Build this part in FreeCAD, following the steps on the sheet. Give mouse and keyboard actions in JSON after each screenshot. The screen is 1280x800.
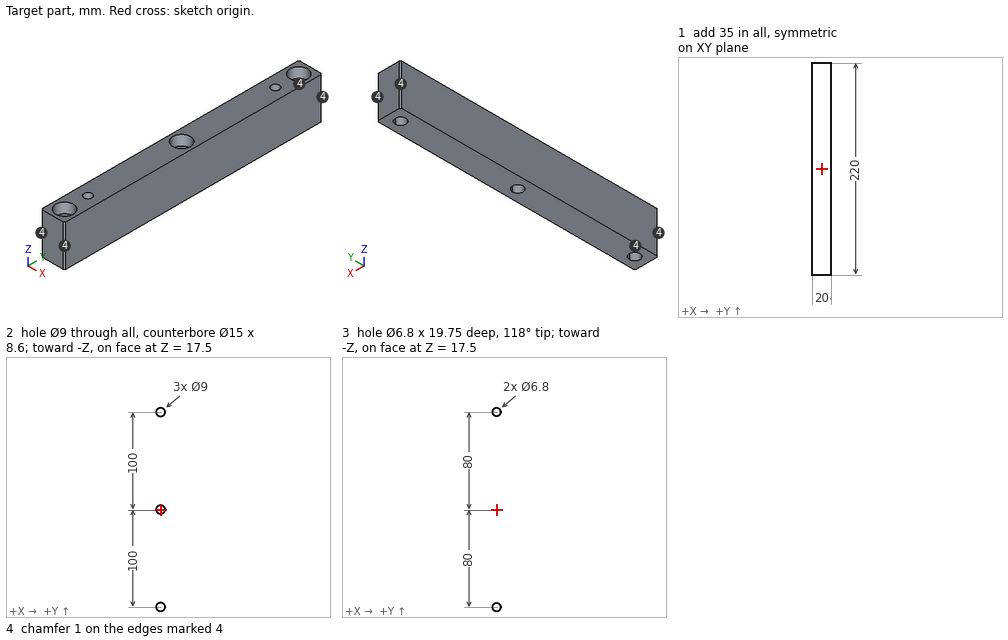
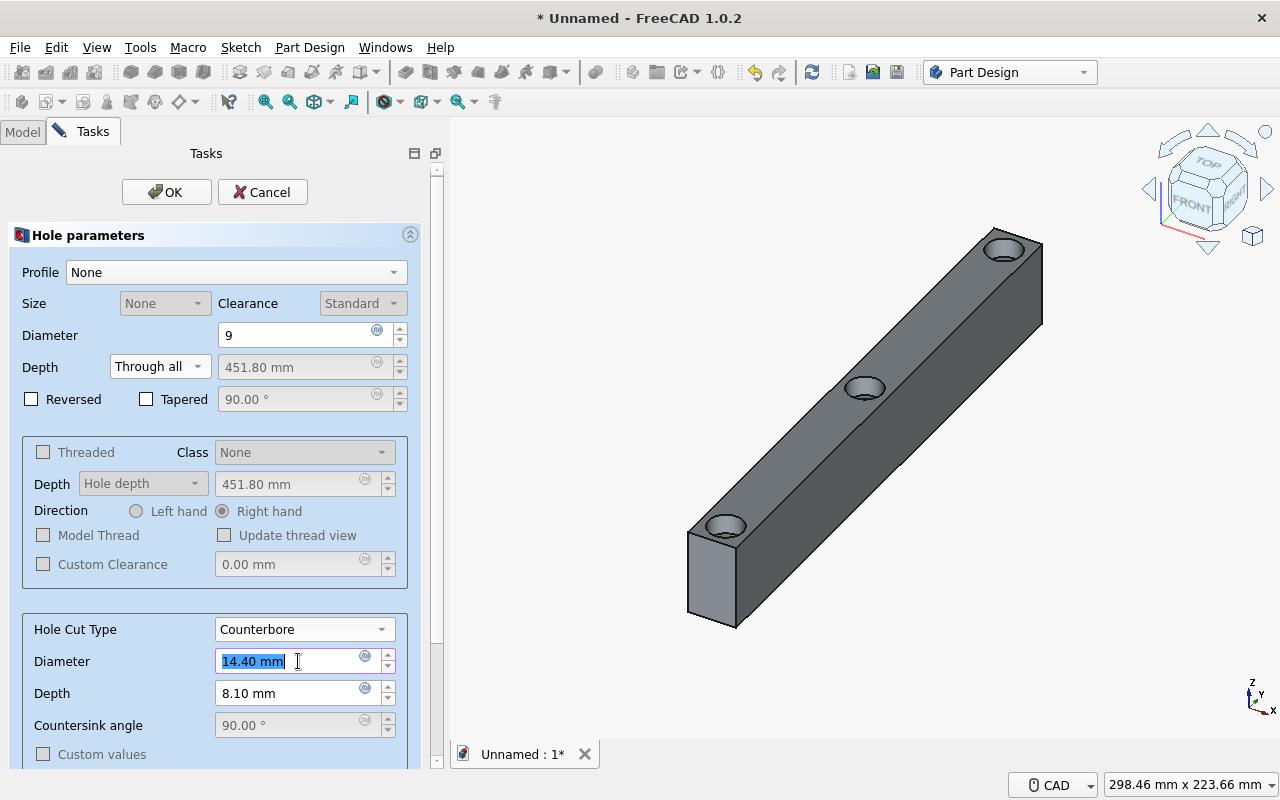
{"action": "type", "text": "15"}
{"action": "key", "text": "Tab"}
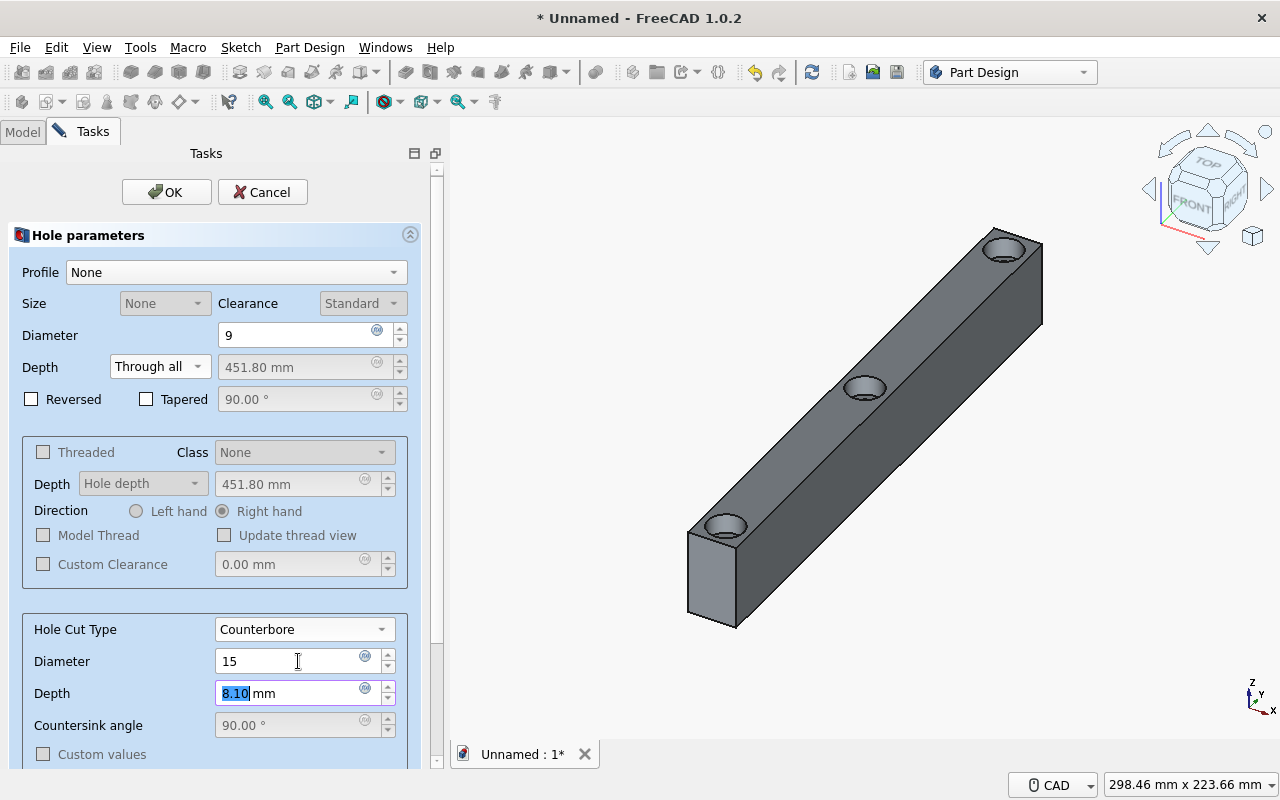
{"action": "type", "text": "8.6"}
{"action": "key", "text": "Tab"}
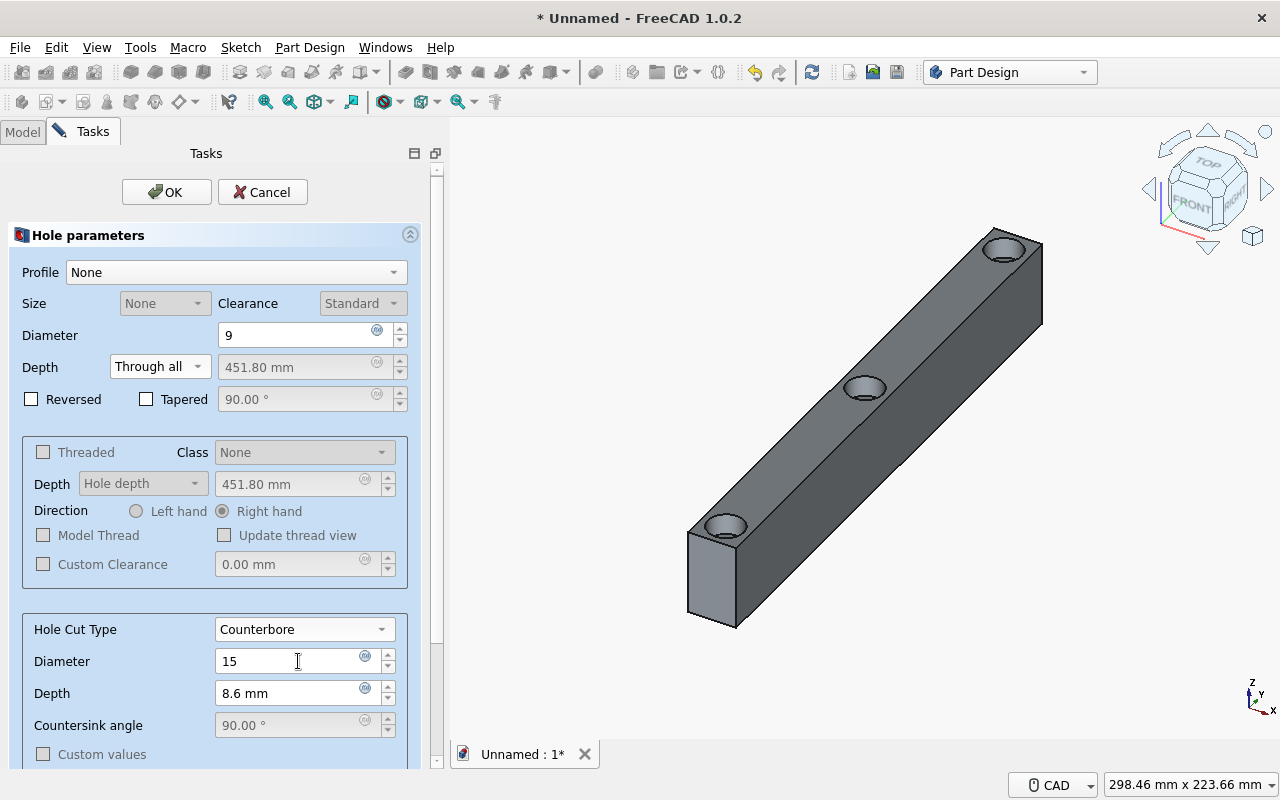
{"action": "left_click", "coordinate": [167, 192]}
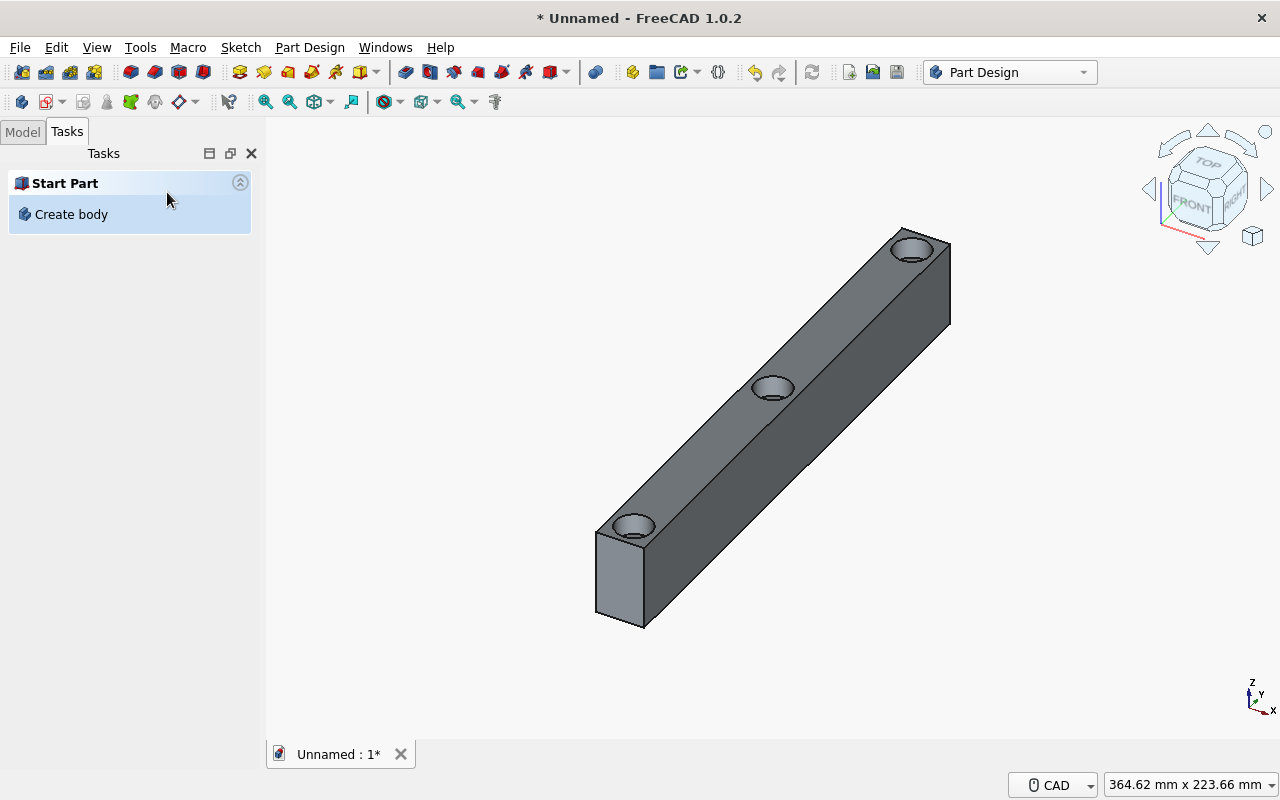
{"action": "left_click", "coordinate": [860, 300]}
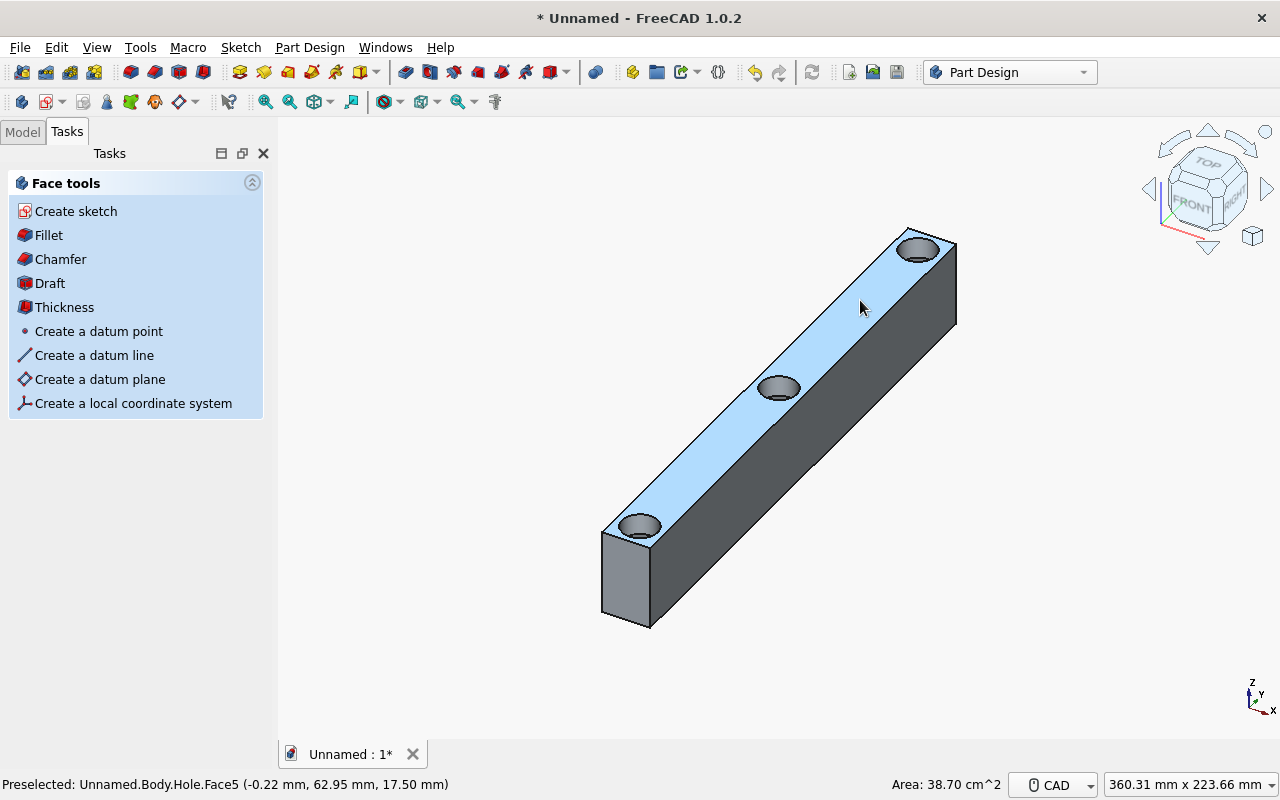
{"action": "left_click", "coordinate": [46, 102]}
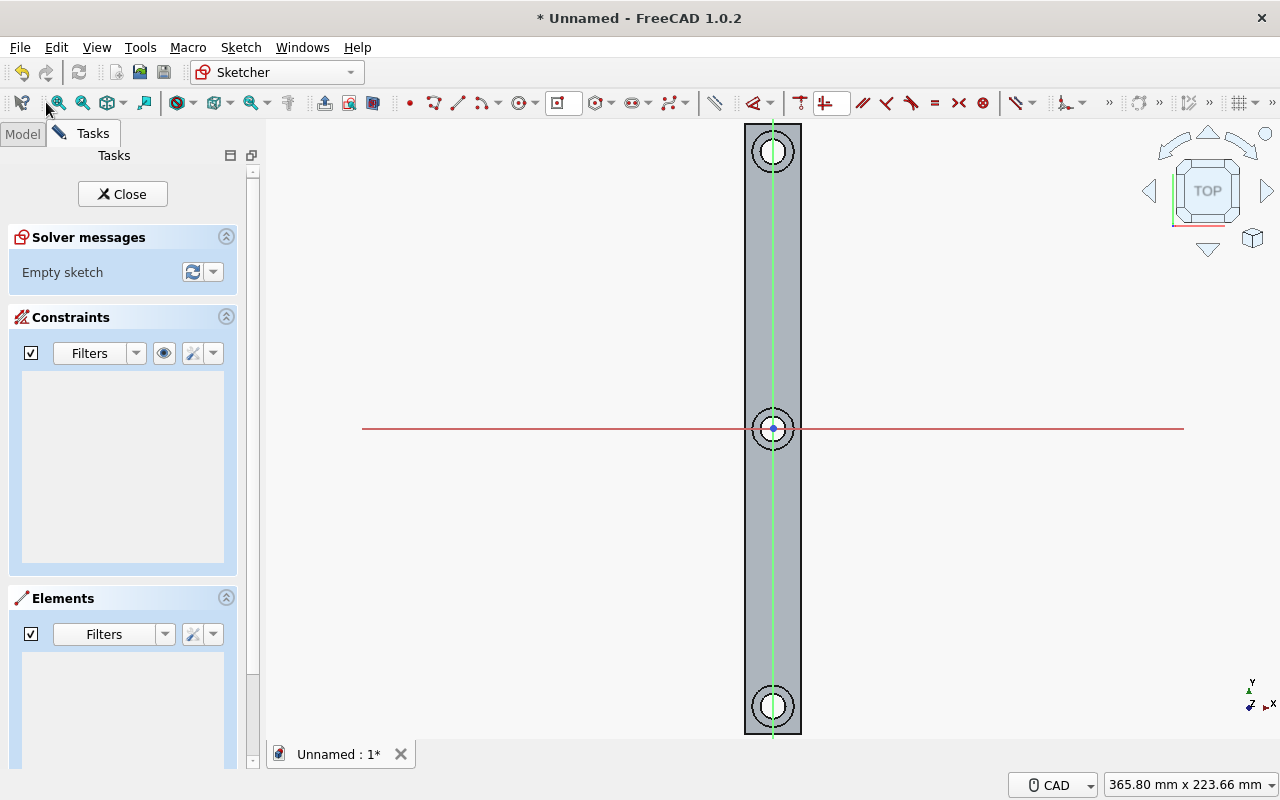
{"action": "left_click", "coordinate": [520, 104]}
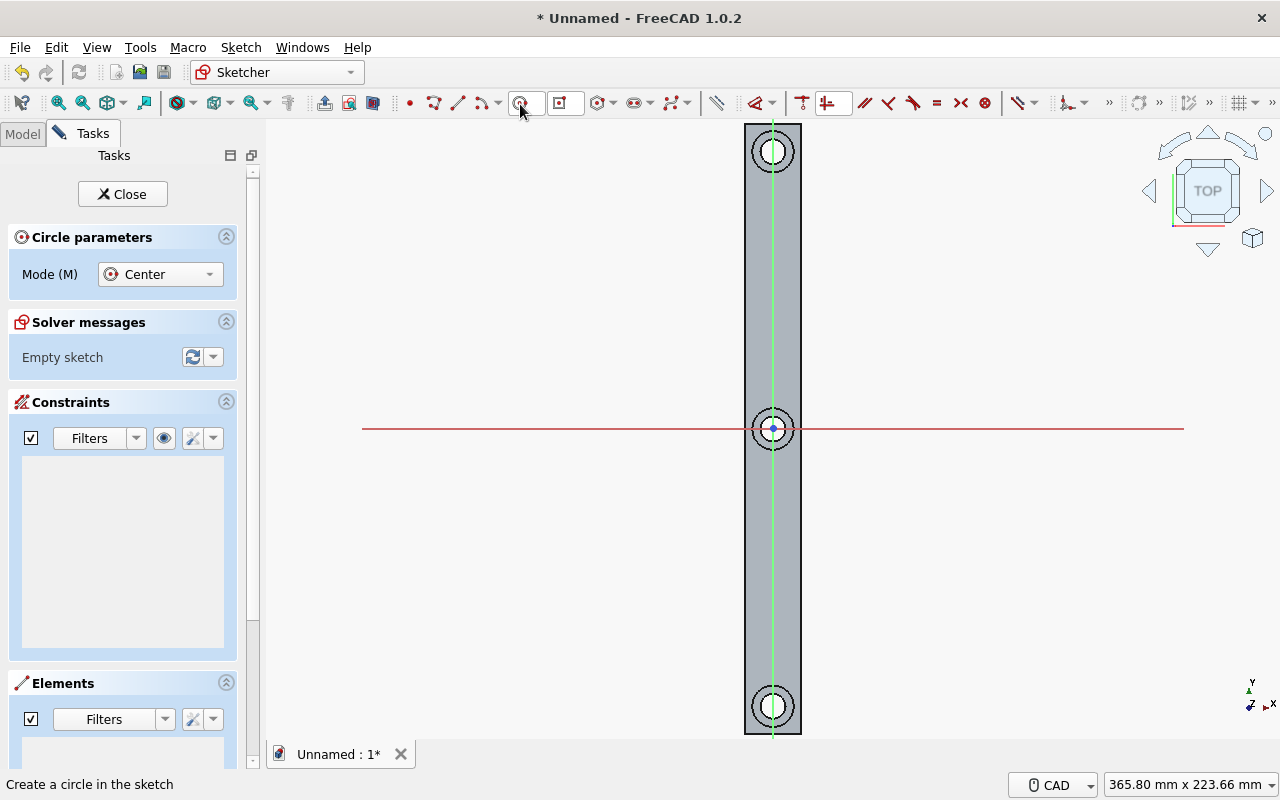
{"action": "scroll", "coordinate": [773, 207], "scroll_direction": "up", "scroll_amount": 5}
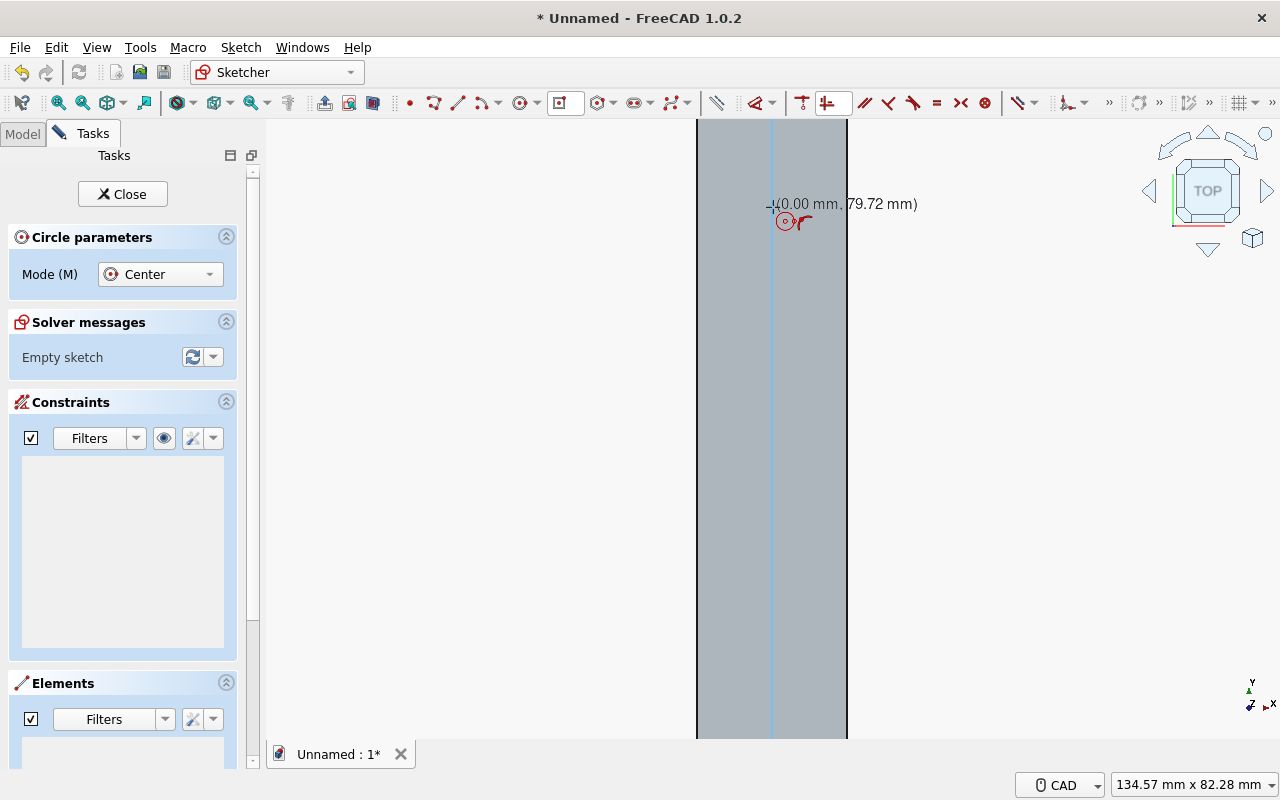
{"action": "left_click", "coordinate": [772, 207]}
{"action": "left_click", "coordinate": [790, 189]}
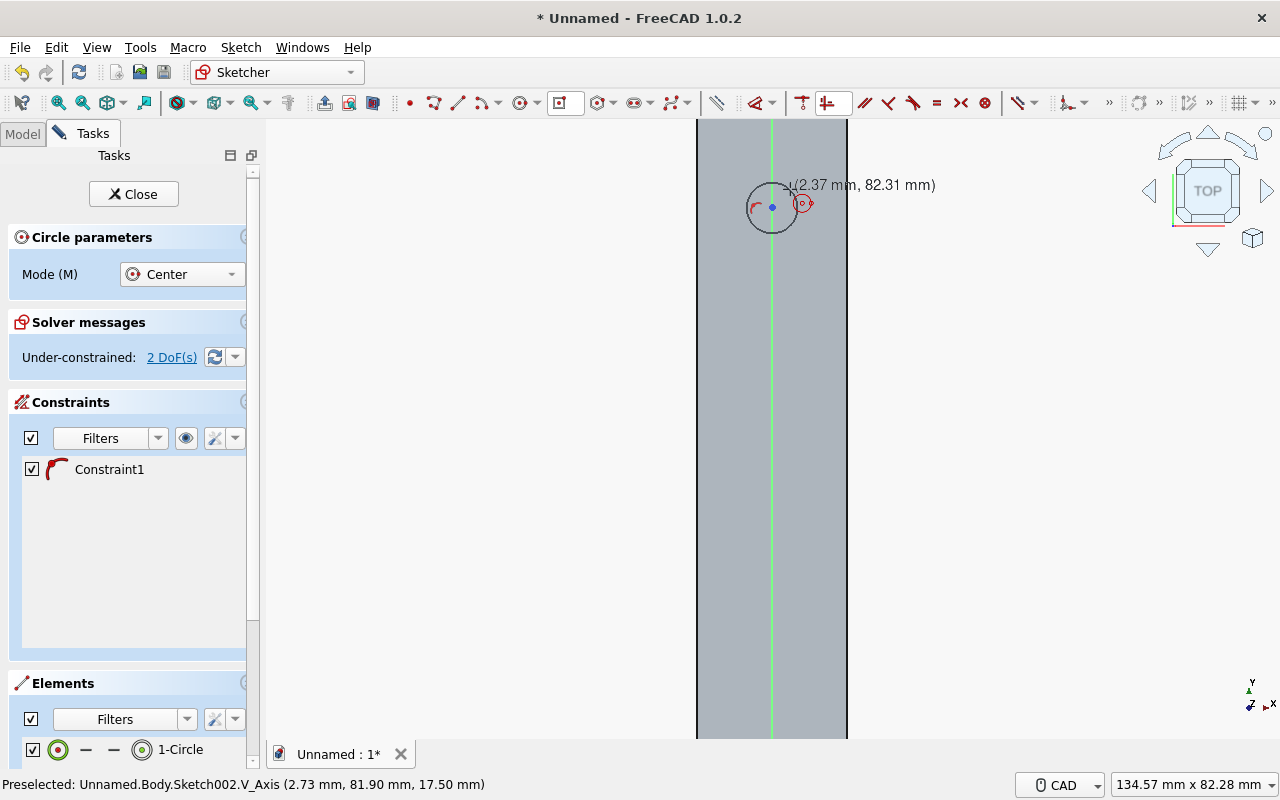
{"action": "scroll", "coordinate": [675, 265], "scroll_direction": "down", "scroll_amount": 6}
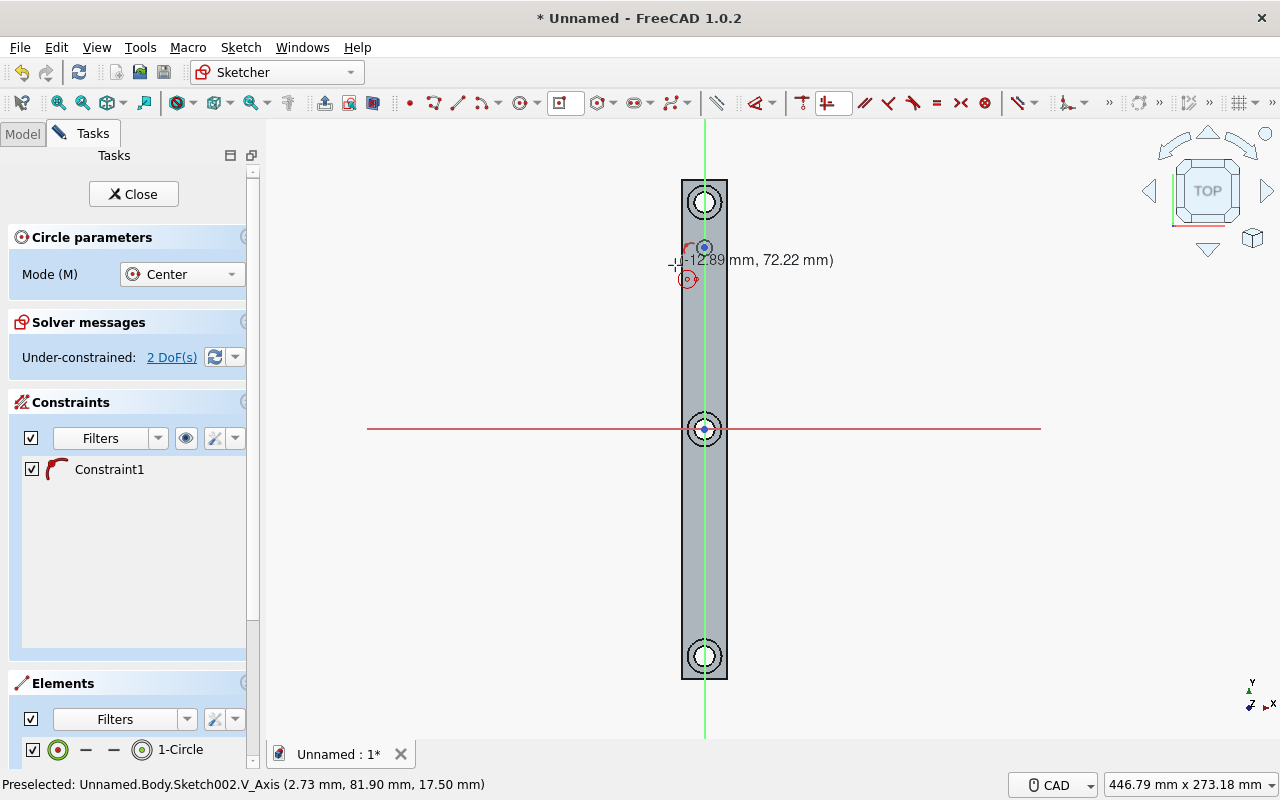
{"action": "scroll", "coordinate": [705, 611], "scroll_direction": "up", "scroll_amount": 6}